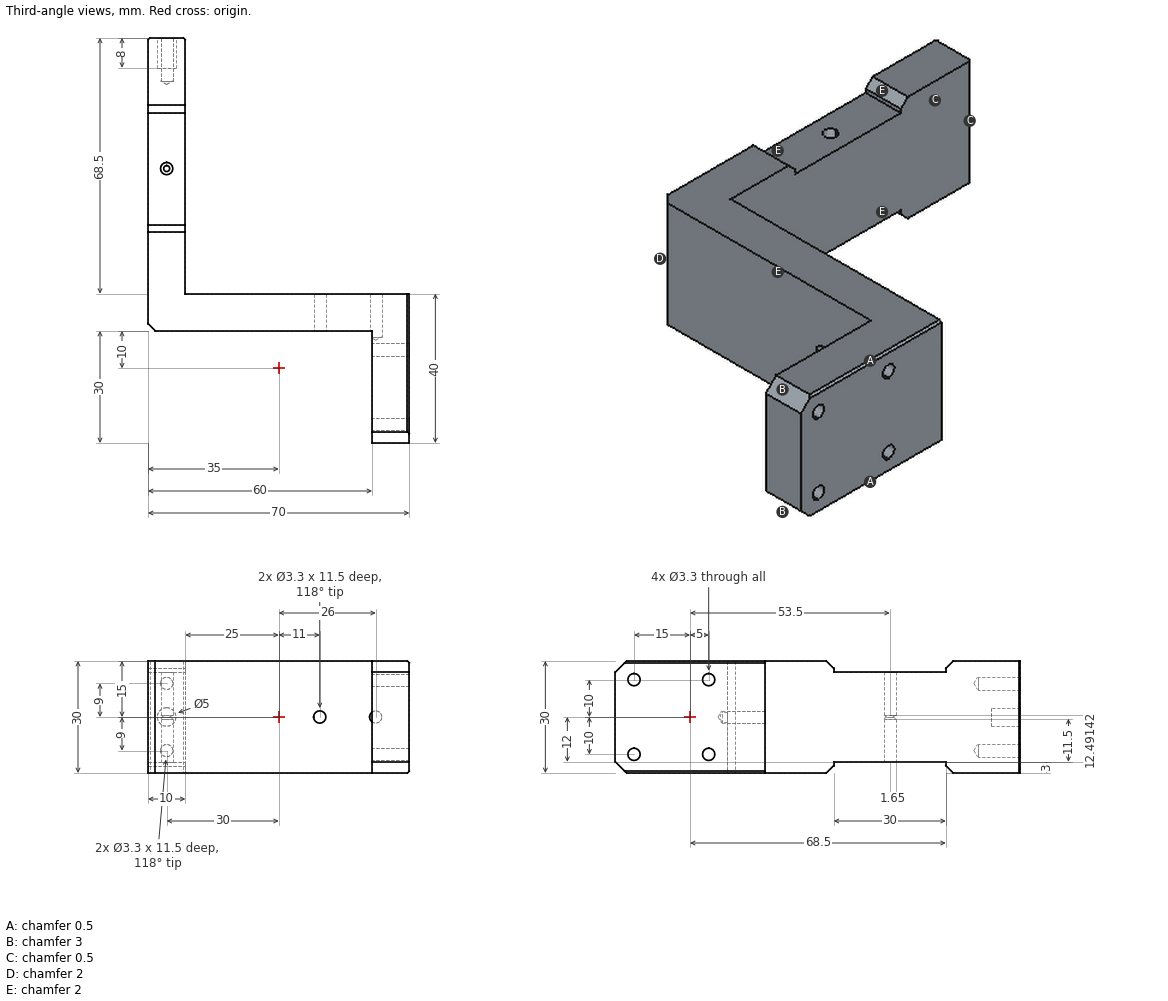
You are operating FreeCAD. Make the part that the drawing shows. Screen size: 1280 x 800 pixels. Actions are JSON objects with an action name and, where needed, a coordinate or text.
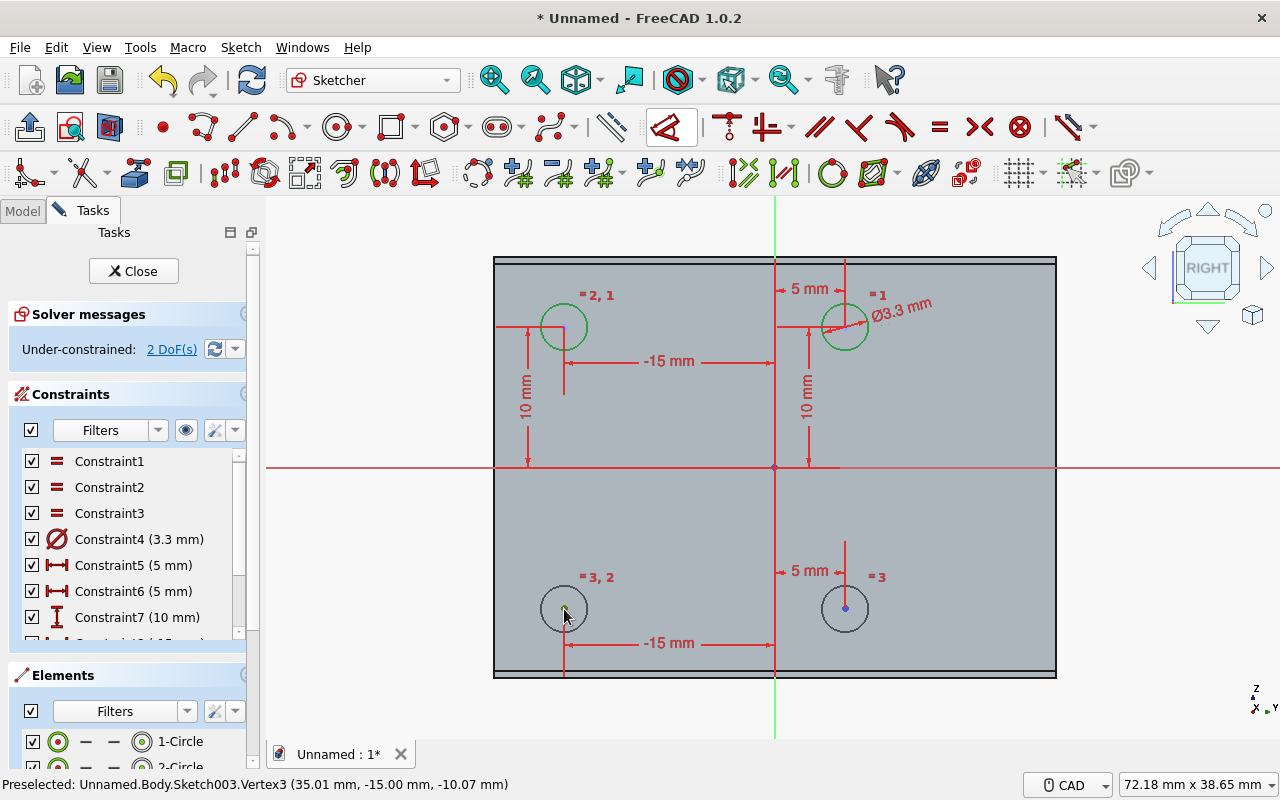
{"action": "left_click", "coordinate": [692, 128]}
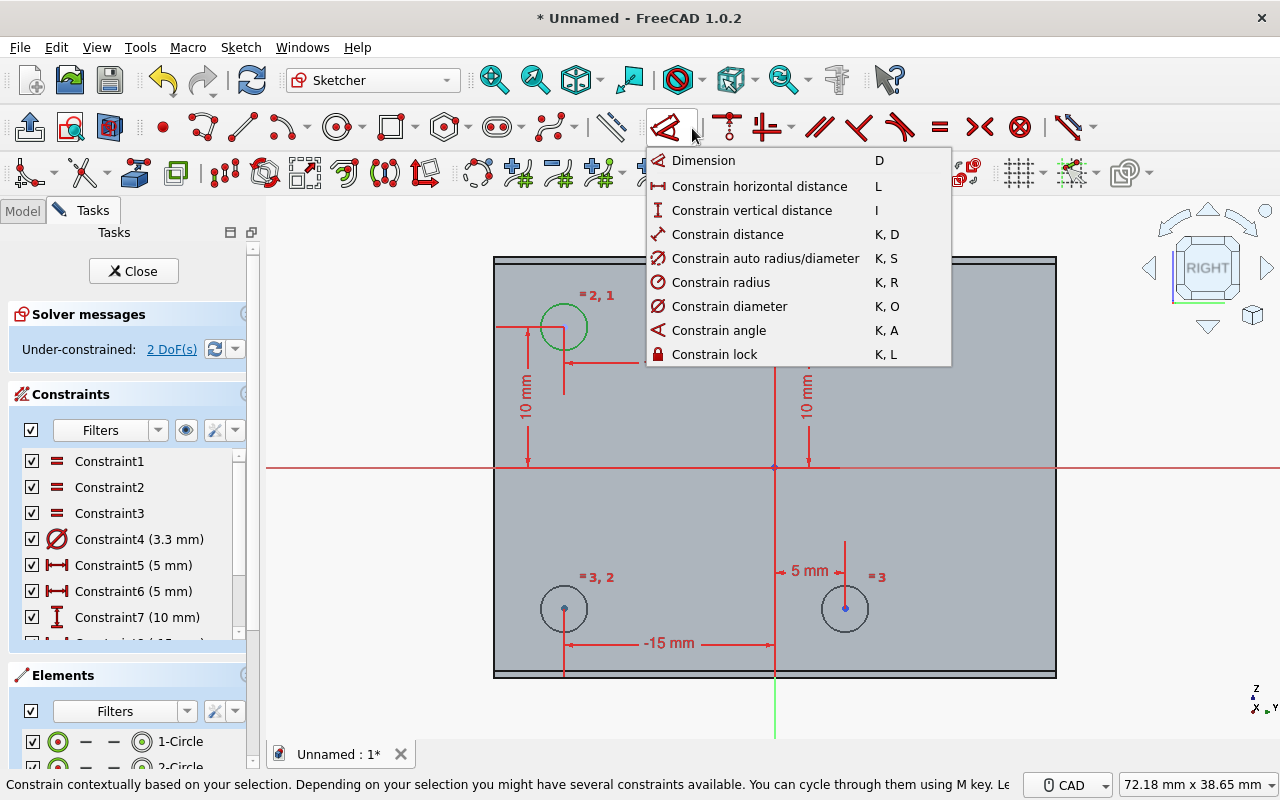
{"action": "left_click", "coordinate": [799, 210]}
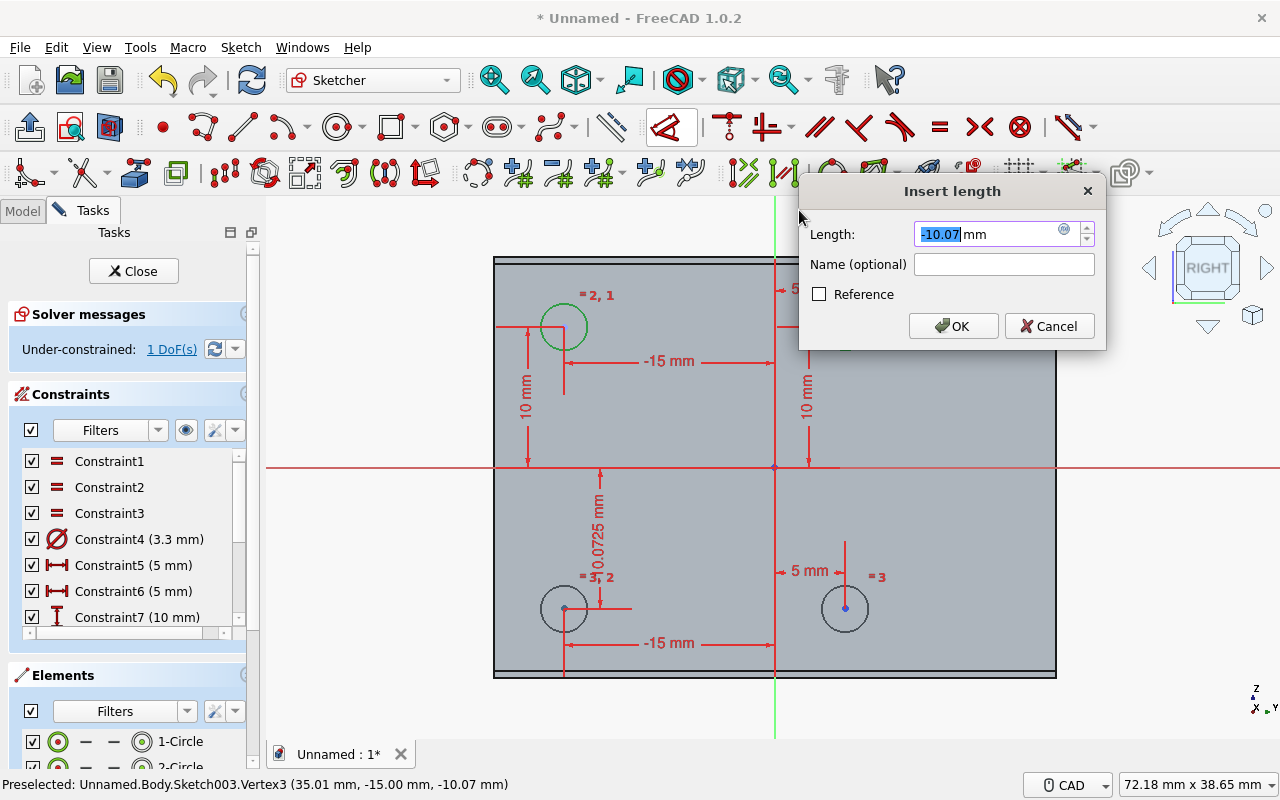
{"action": "type", "text": "-10"}
{"action": "key", "text": "Return"}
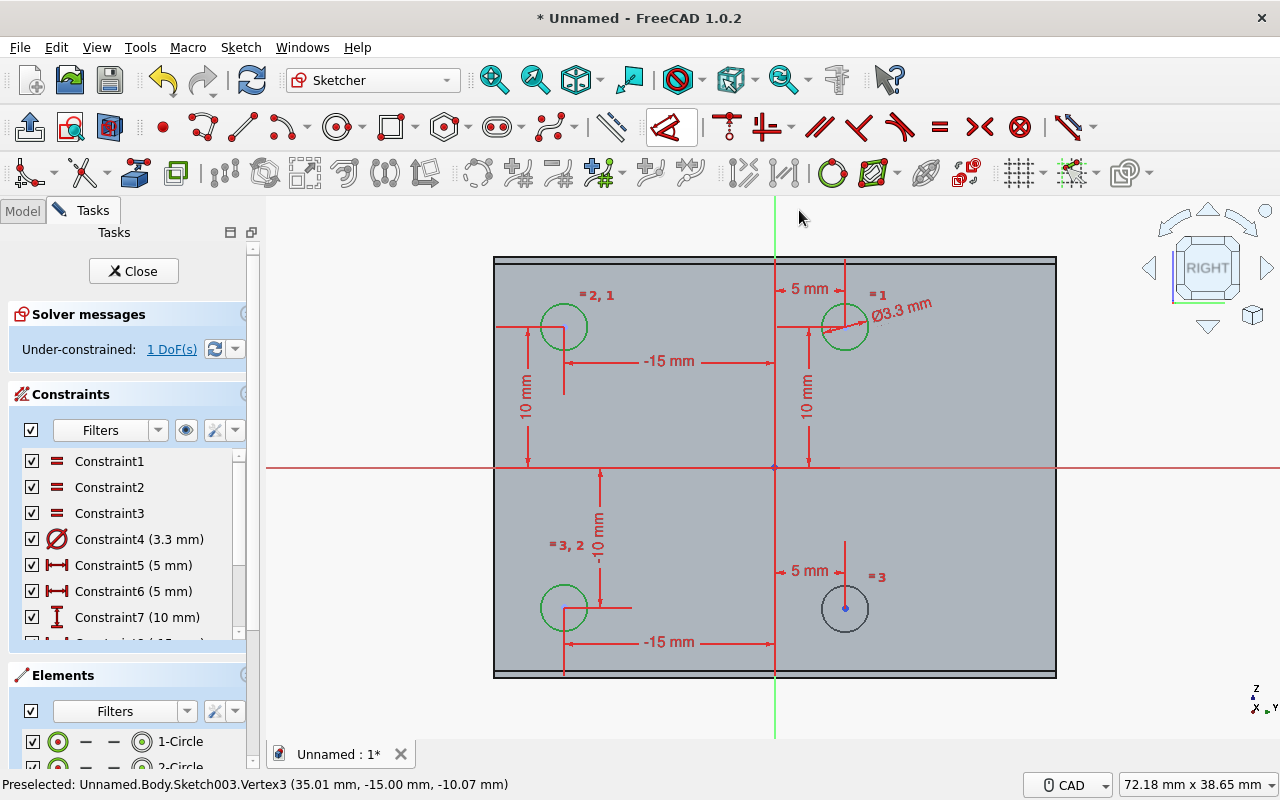
{"action": "left_click", "coordinate": [845, 609]}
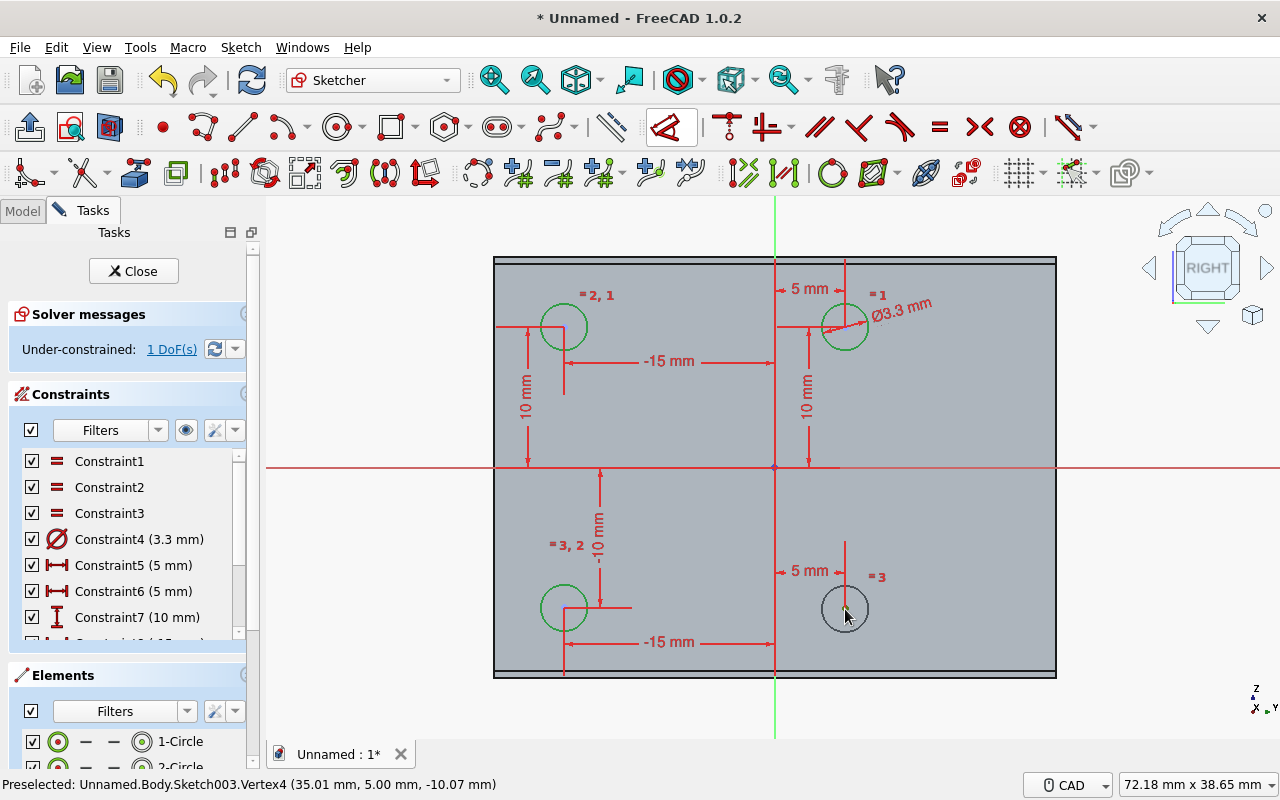
{"action": "left_click", "coordinate": [692, 128]}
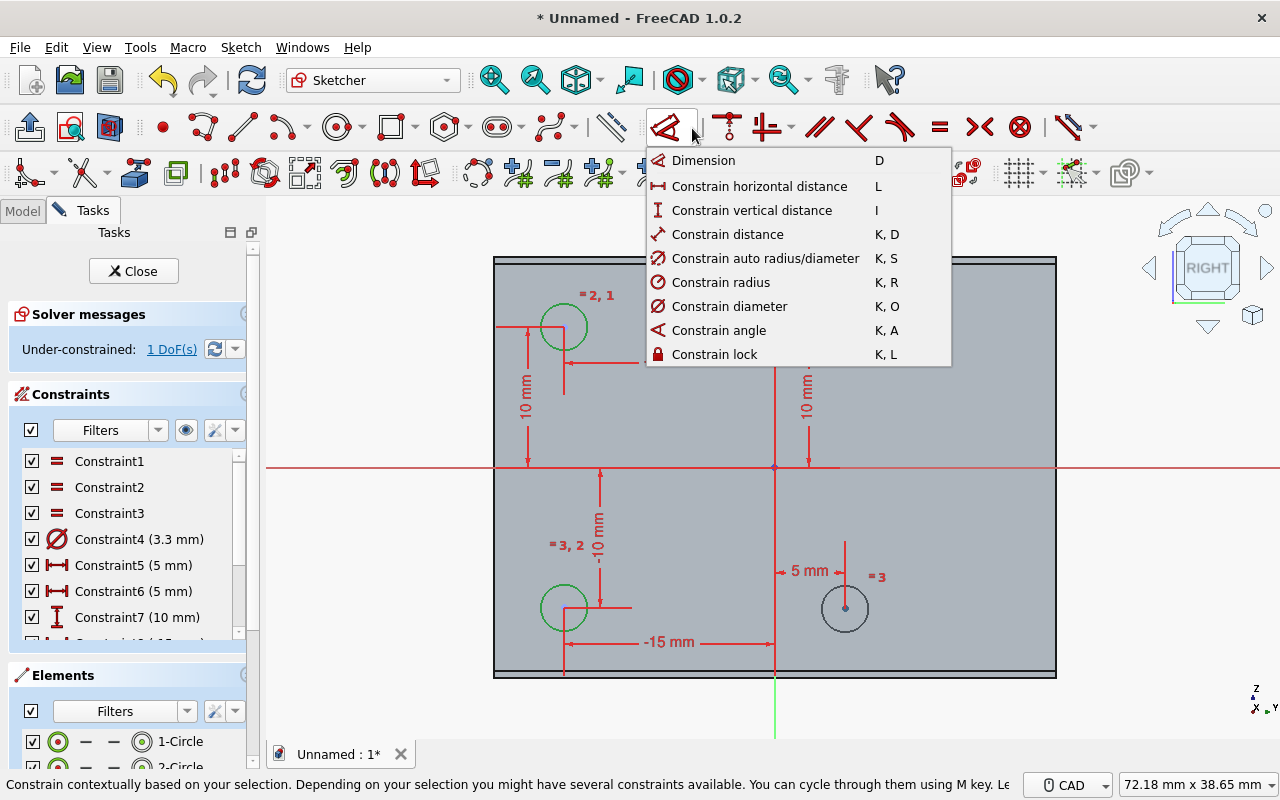
{"action": "left_click", "coordinate": [799, 210]}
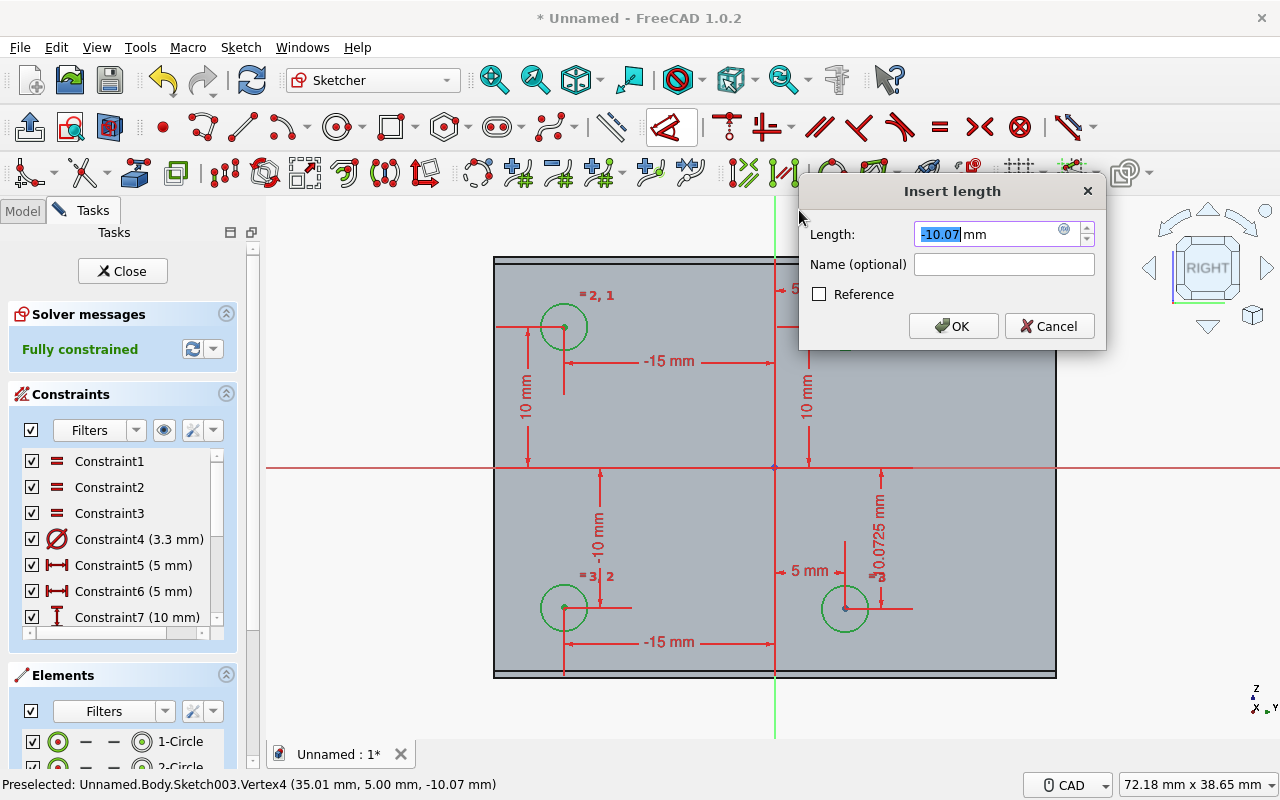
{"action": "type", "text": "-10"}
{"action": "key", "text": "Return"}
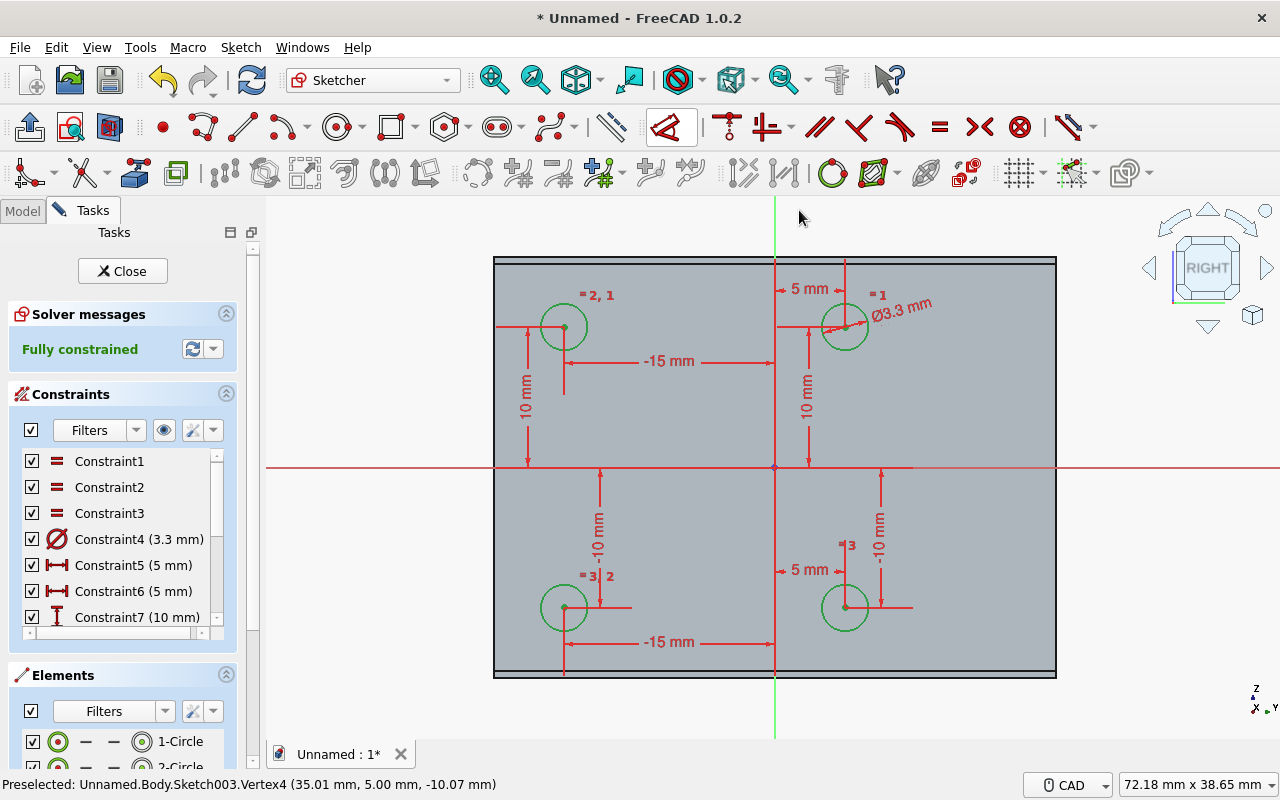
{"action": "left_click", "coordinate": [123, 271]}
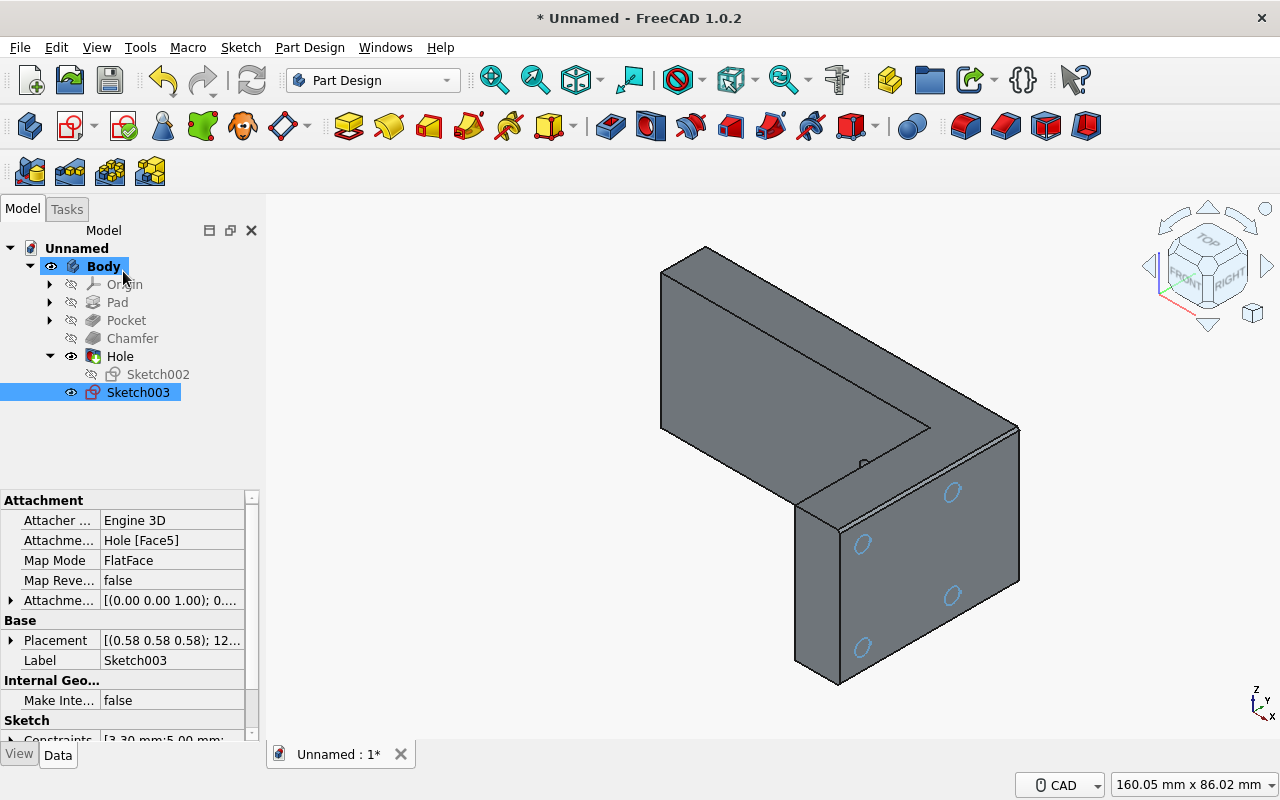
{"action": "left_click", "coordinate": [652, 126]}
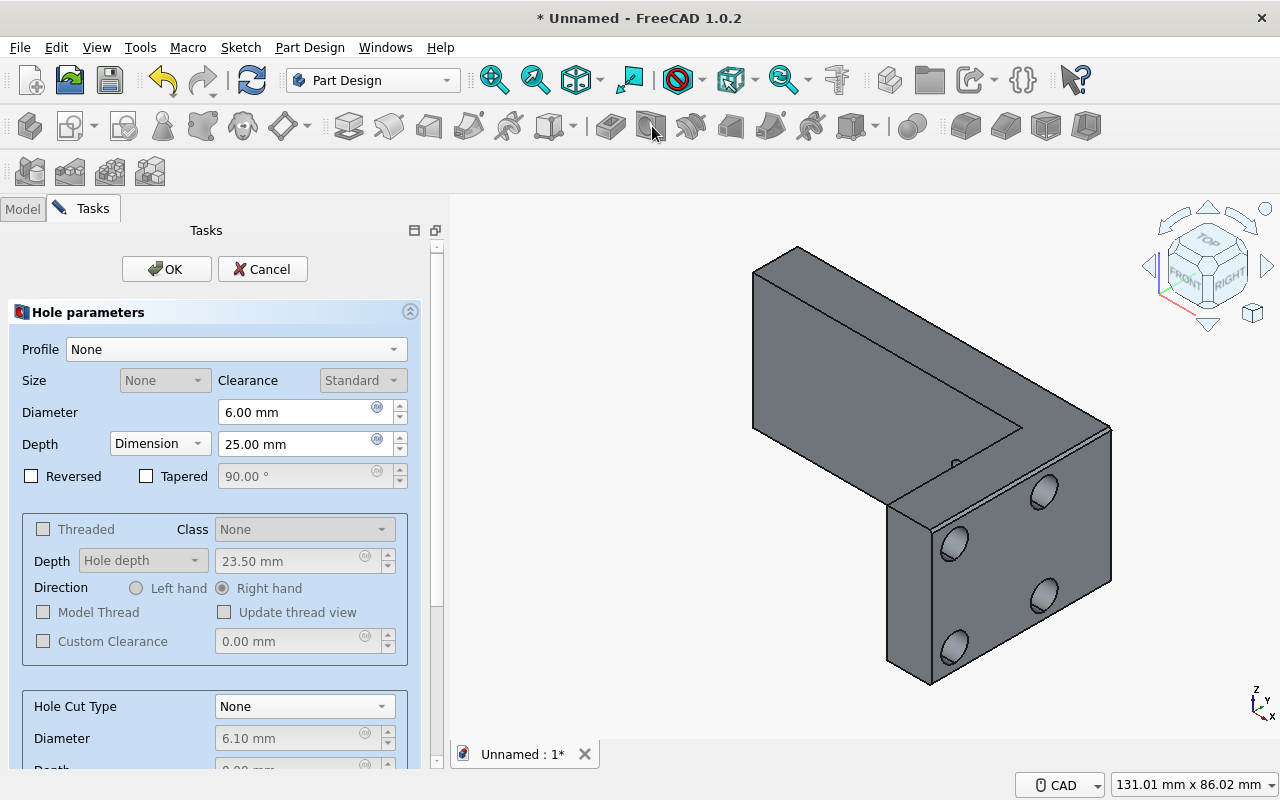
{"action": "triple_click", "coordinate": [305, 412]}